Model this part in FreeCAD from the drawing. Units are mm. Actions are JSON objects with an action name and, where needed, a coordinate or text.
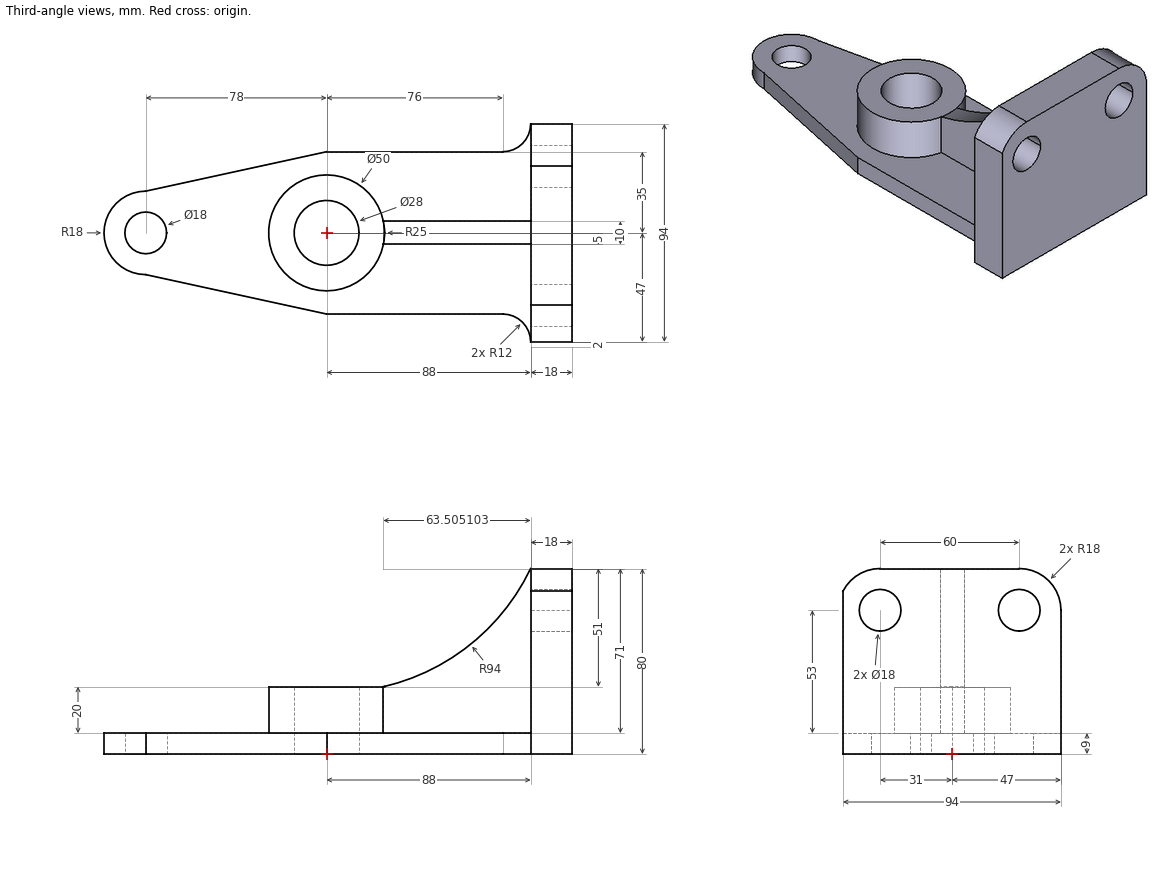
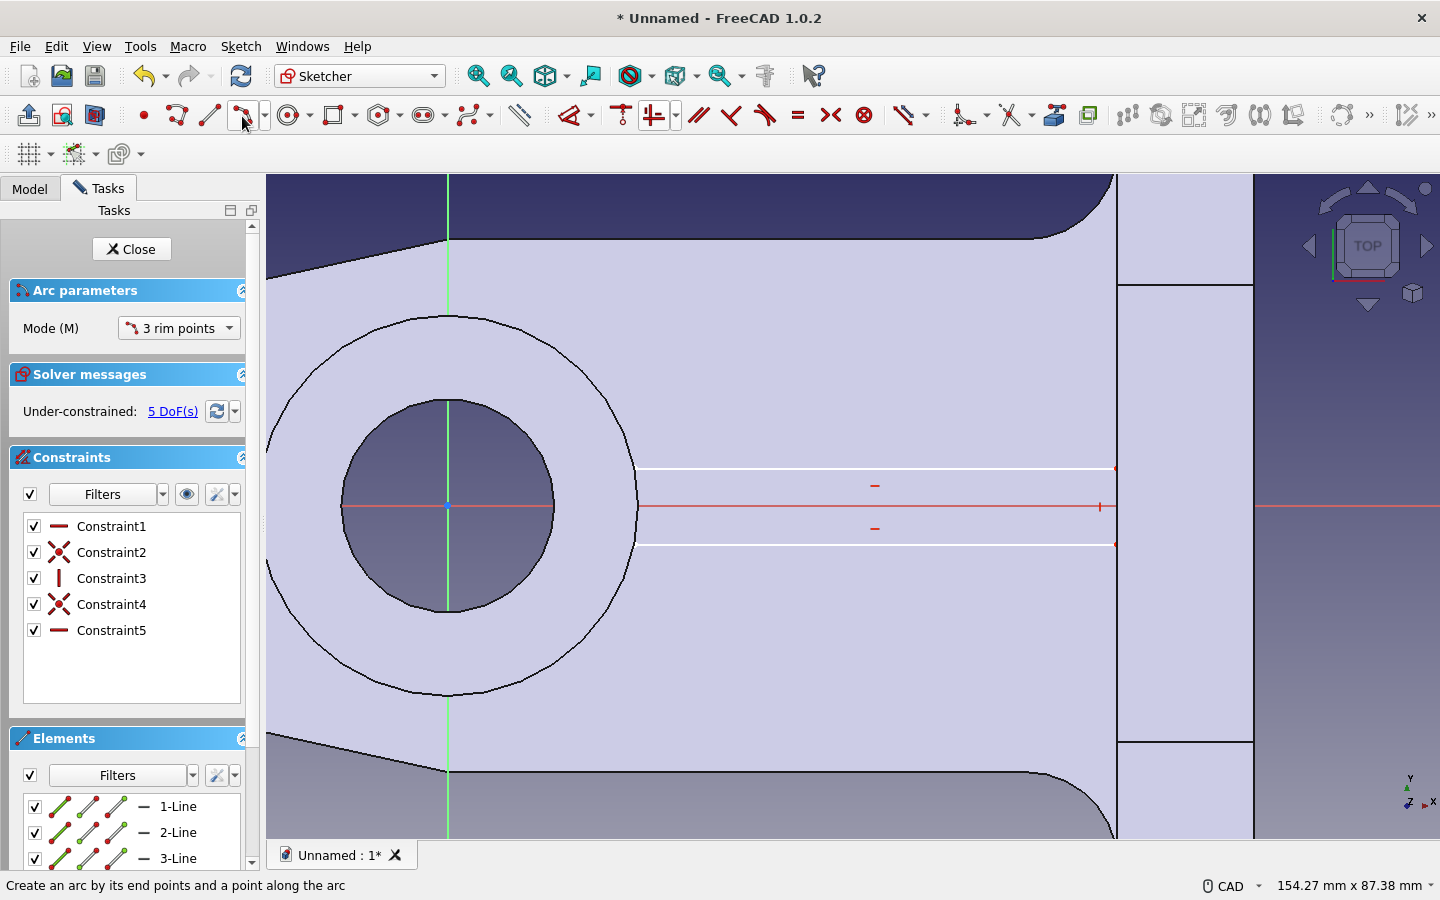
{"action": "left_click", "coordinate": [634, 469]}
{"action": "left_click", "coordinate": [634, 545]}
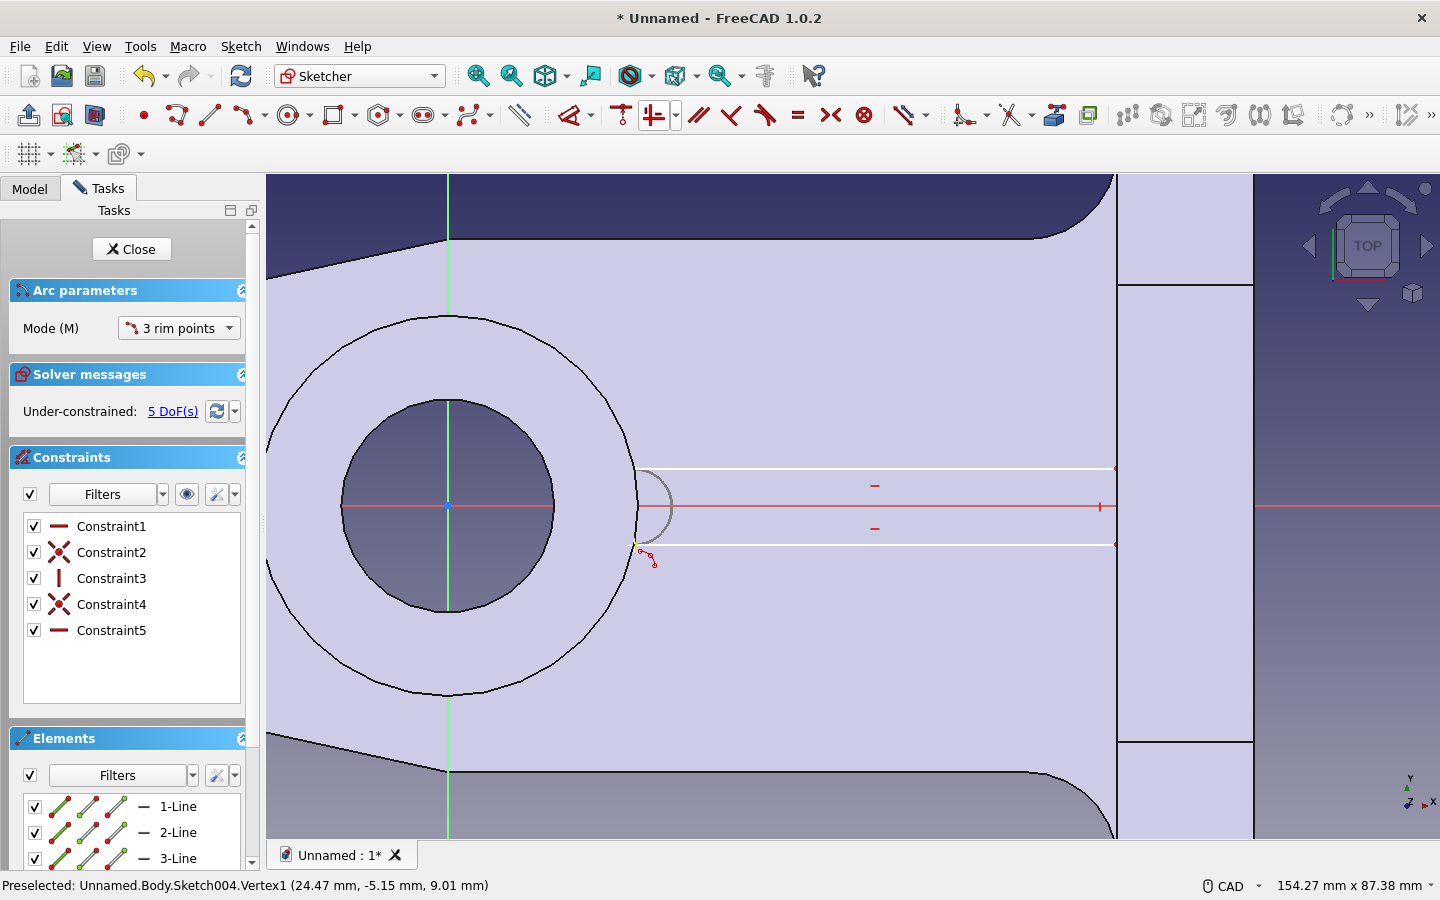
{"action": "scroll", "coordinate": [638, 513], "scroll_direction": "up", "scroll_amount": 8}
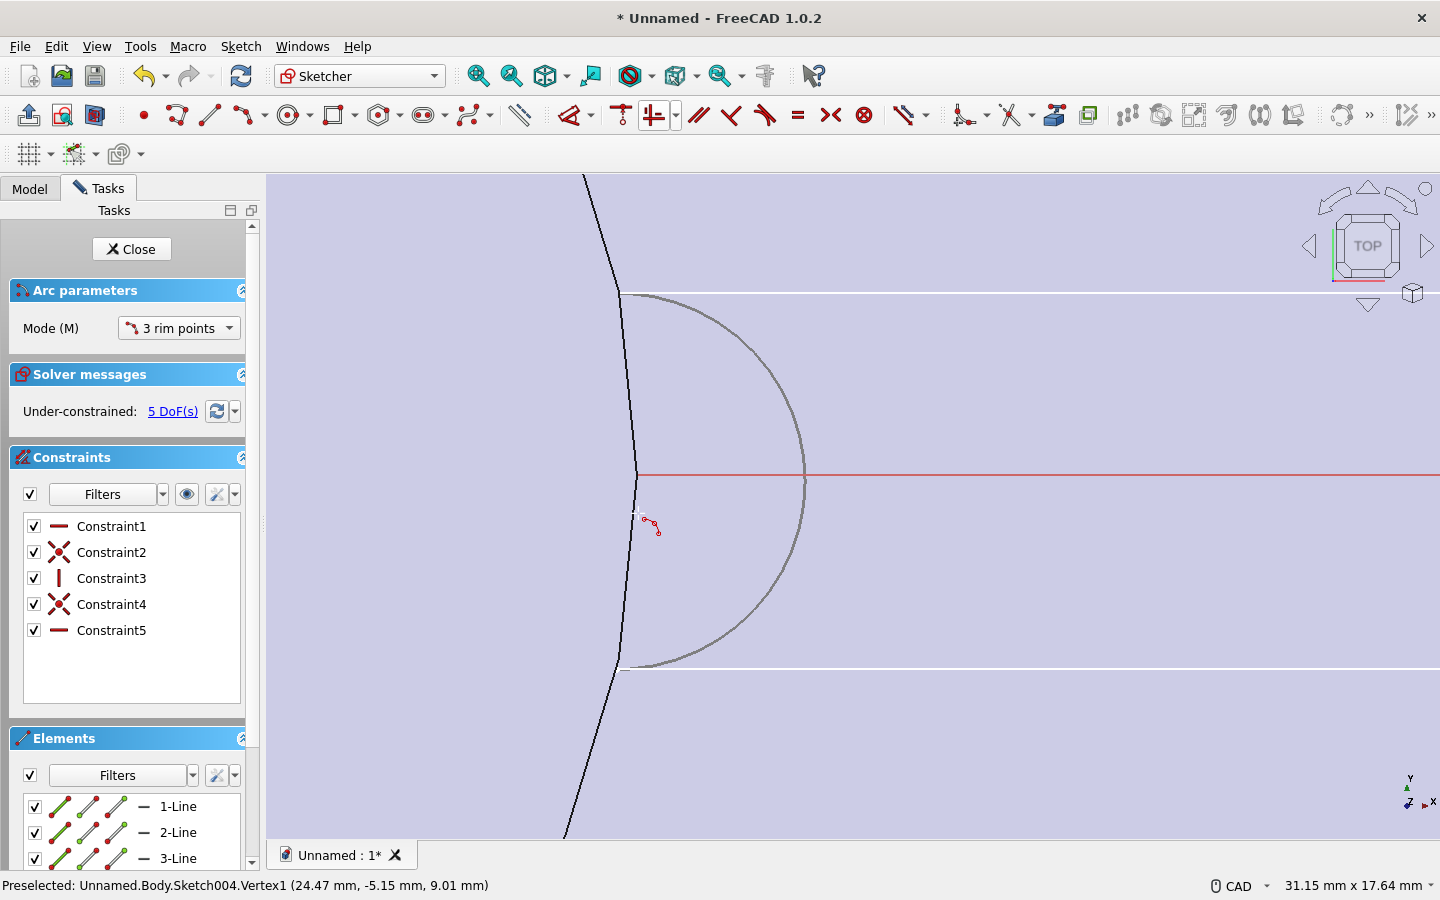
{"action": "left_click", "coordinate": [636, 513]}
{"action": "key", "text": "Escape"}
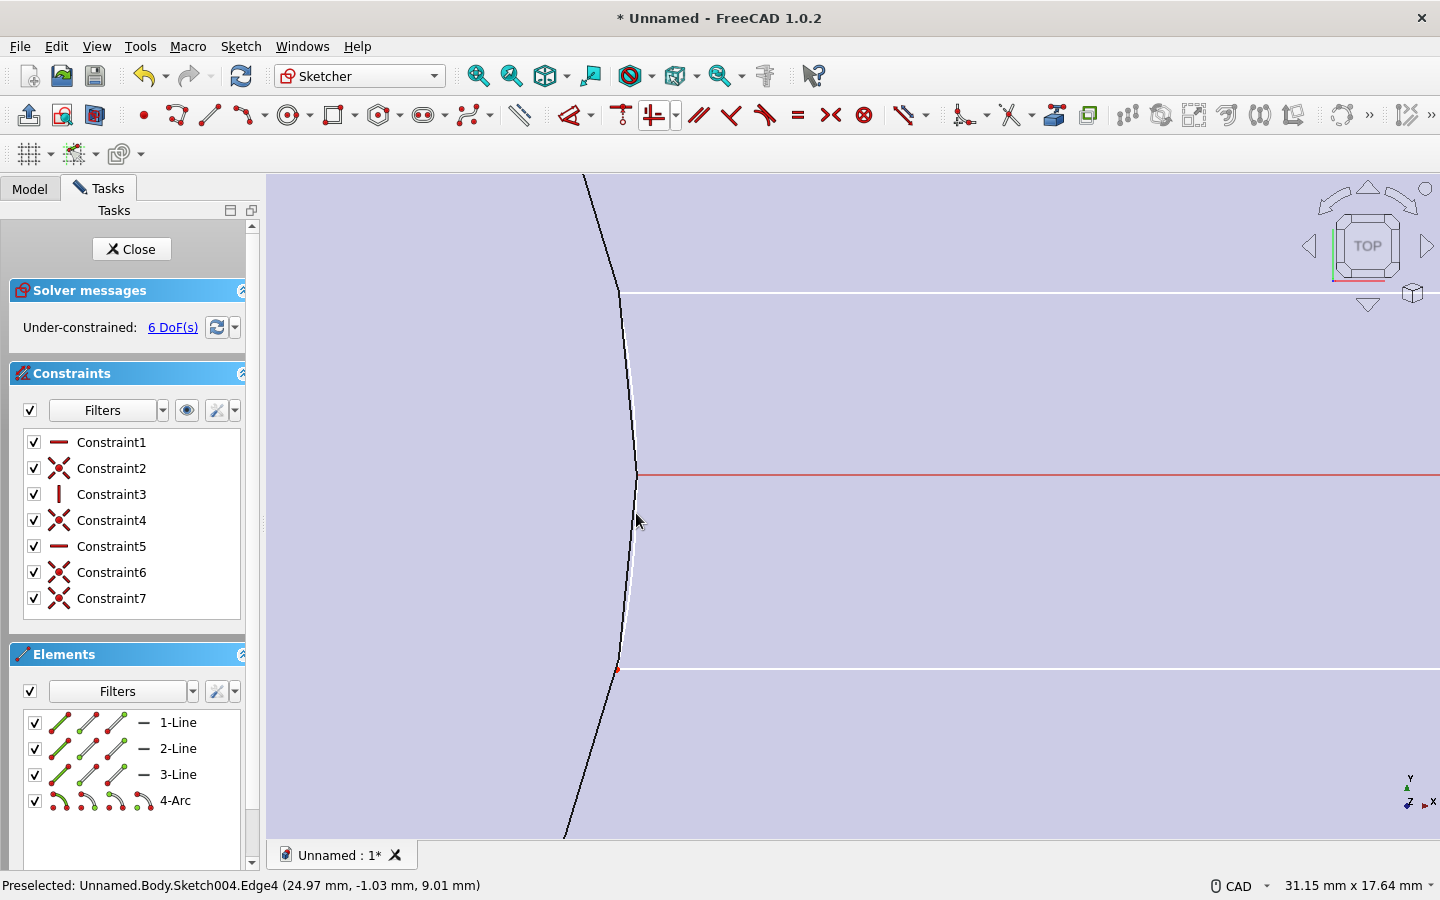
{"action": "scroll", "coordinate": [641, 514], "scroll_direction": "down", "scroll_amount": 8}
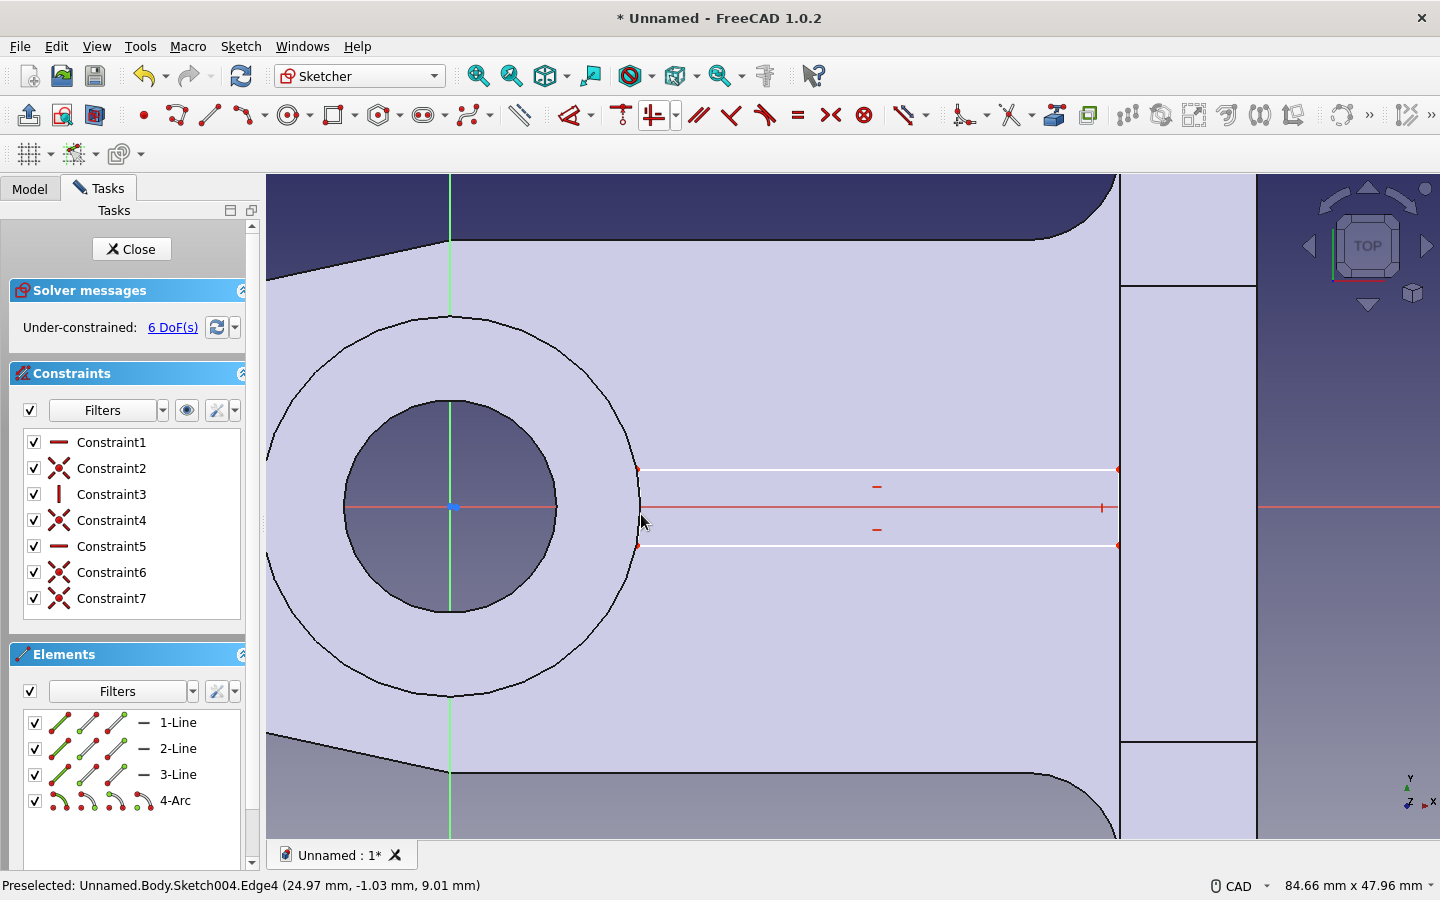
{"action": "left_click_drag", "start_coordinate": [440, 497], "coordinate": [466, 518]}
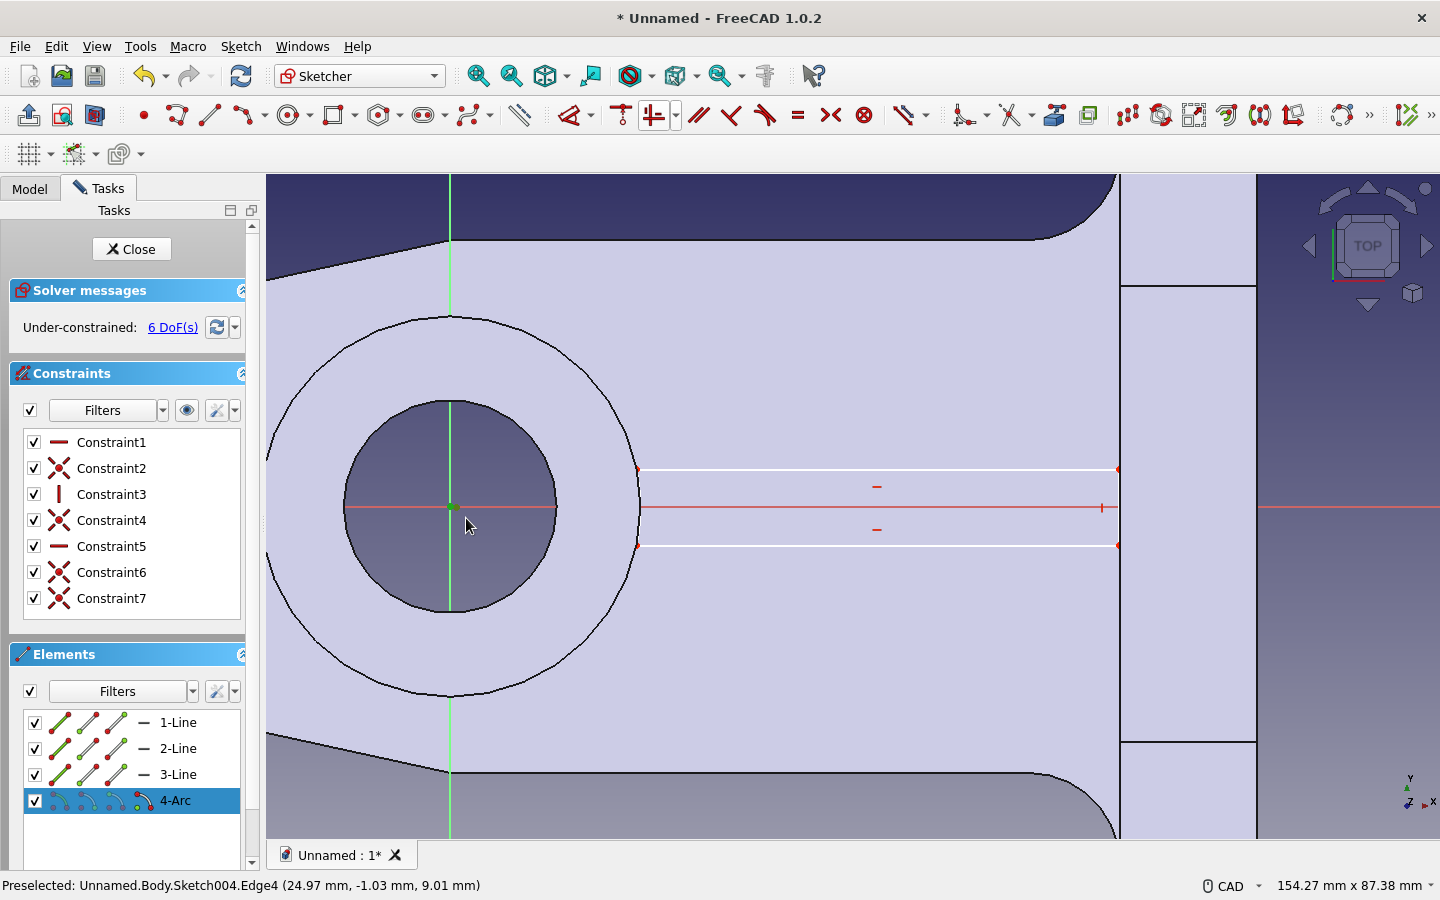
{"action": "left_click", "coordinate": [621, 116]}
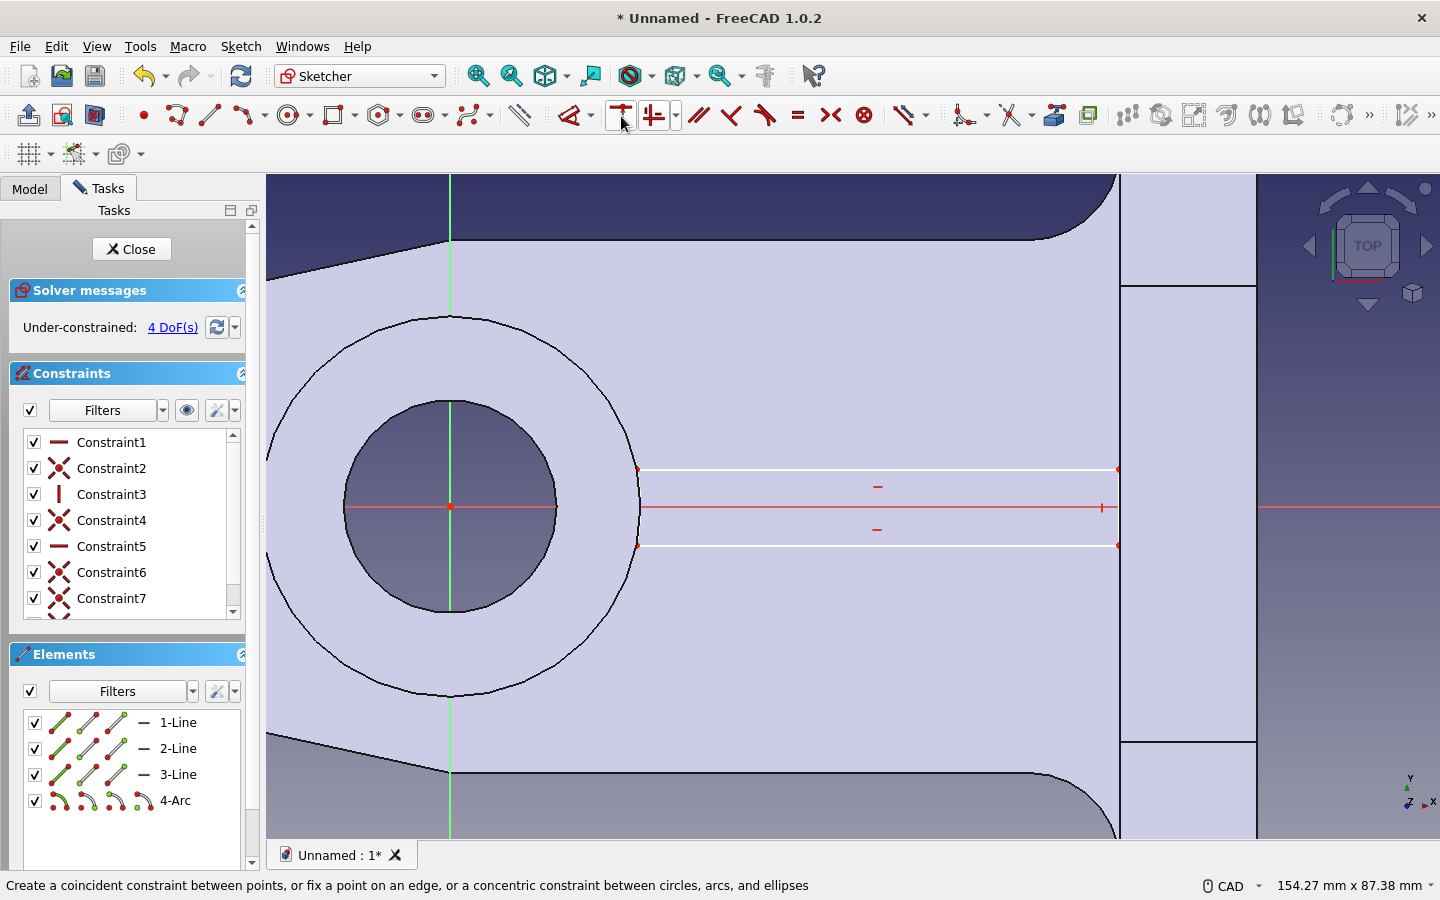
{"action": "left_click", "coordinate": [568, 116]}